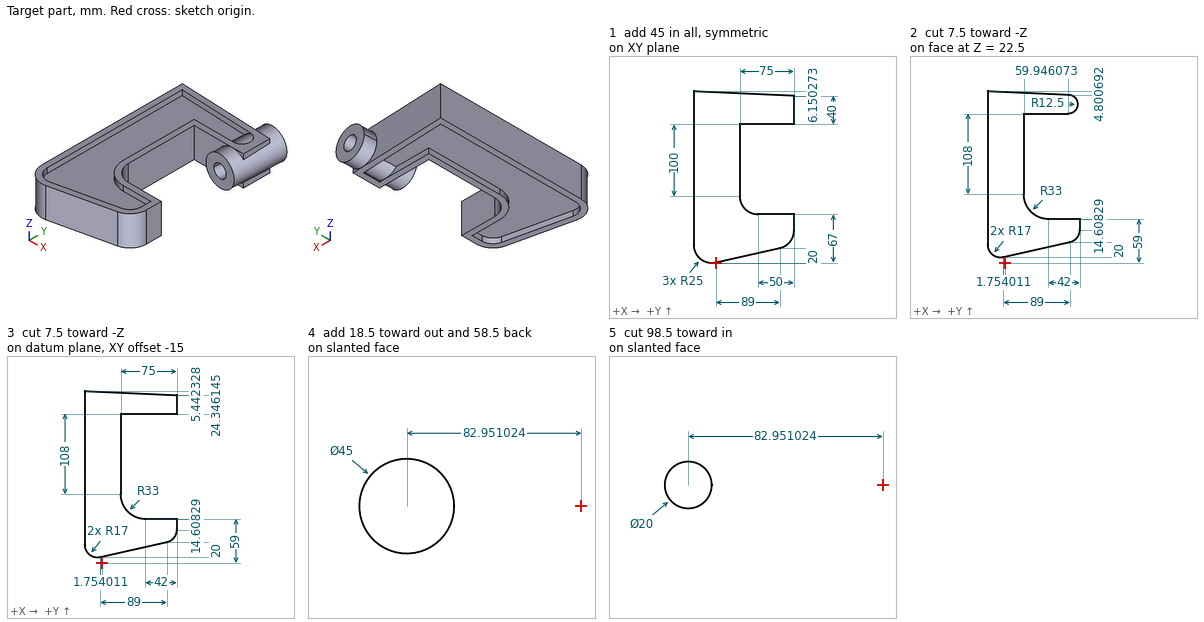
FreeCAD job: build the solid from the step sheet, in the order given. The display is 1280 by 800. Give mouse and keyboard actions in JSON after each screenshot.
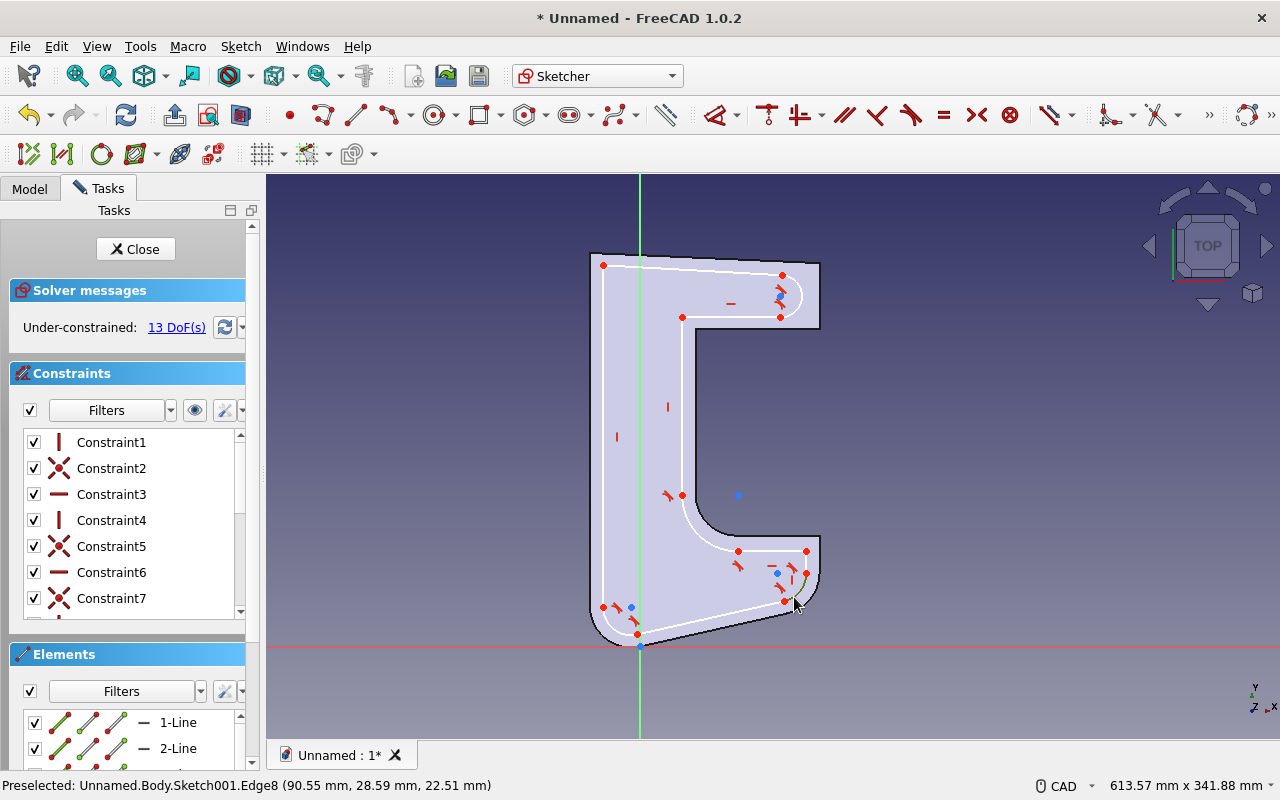
{"action": "left_click", "coordinate": [607, 622]}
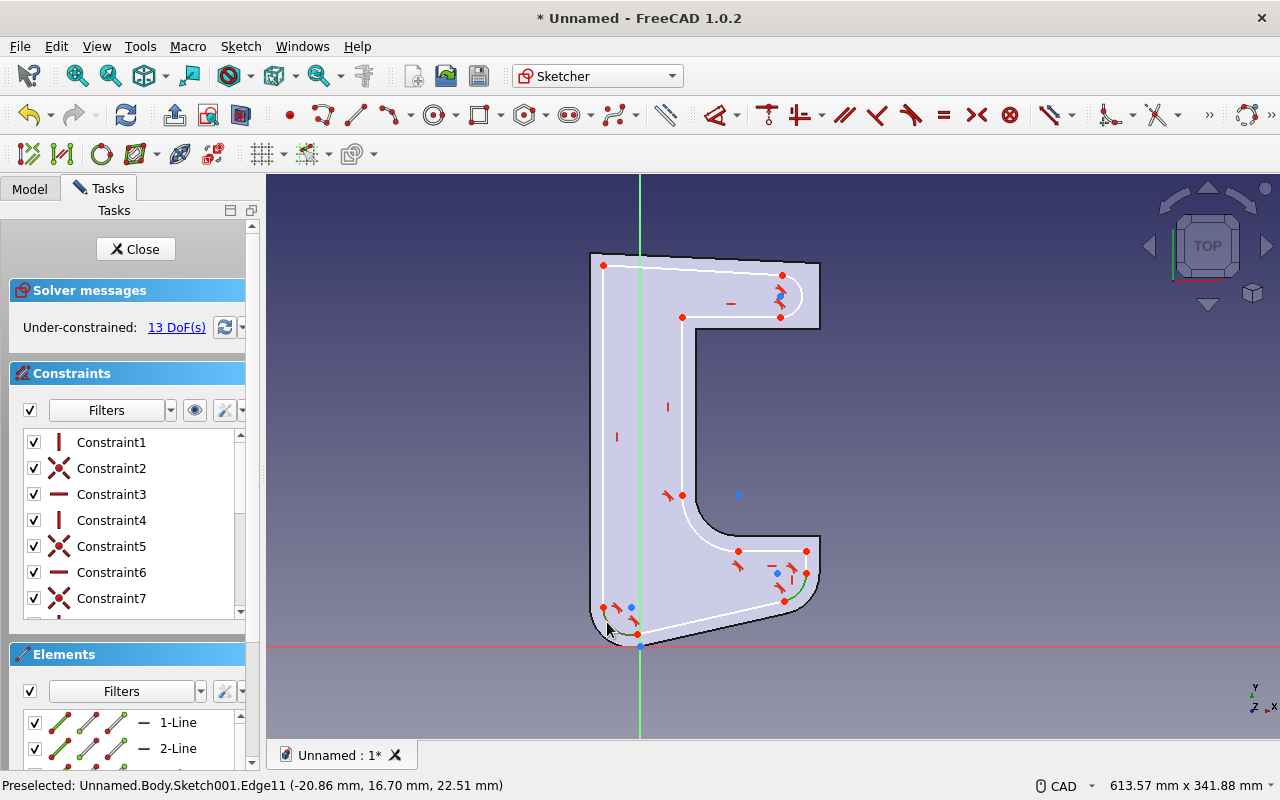
{"action": "left_click", "coordinate": [944, 116]}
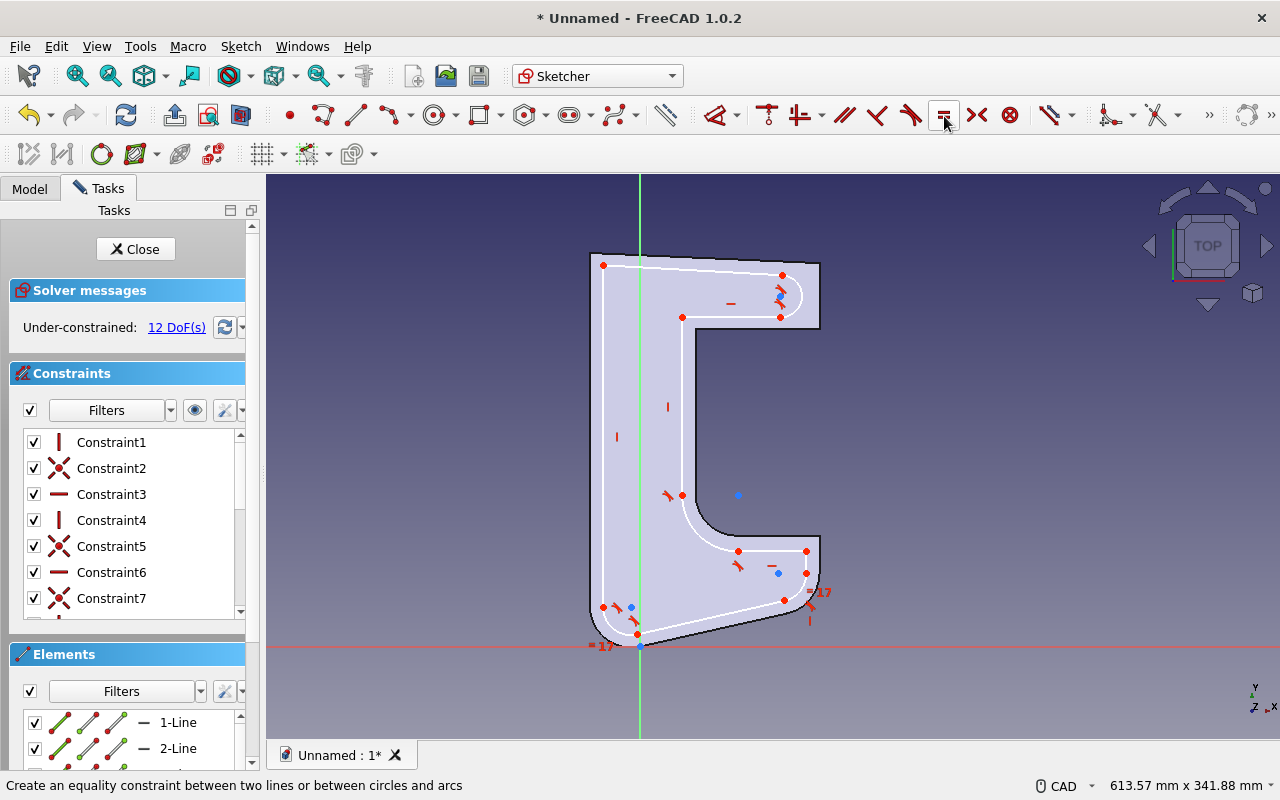
{"action": "left_click", "coordinate": [714, 116]}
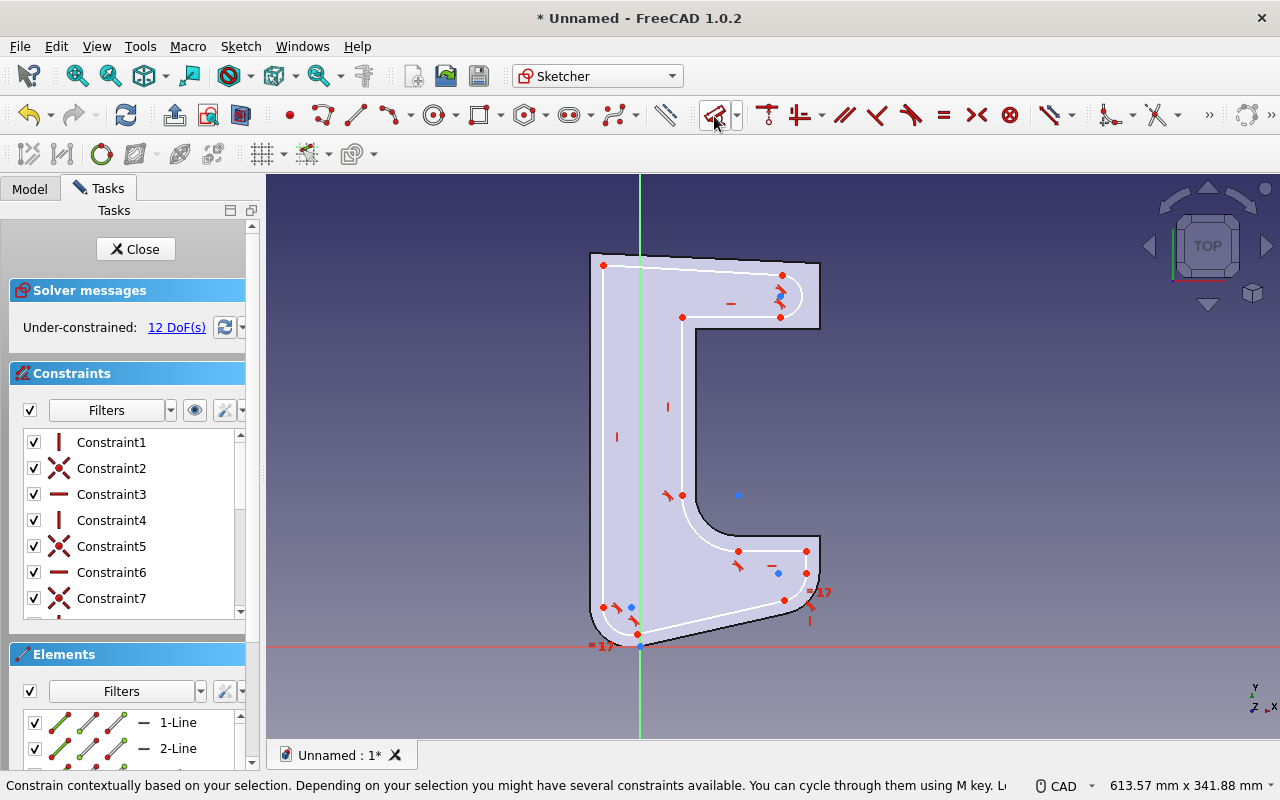
{"action": "scroll", "coordinate": [795, 596], "scroll_direction": "up", "scroll_amount": 2}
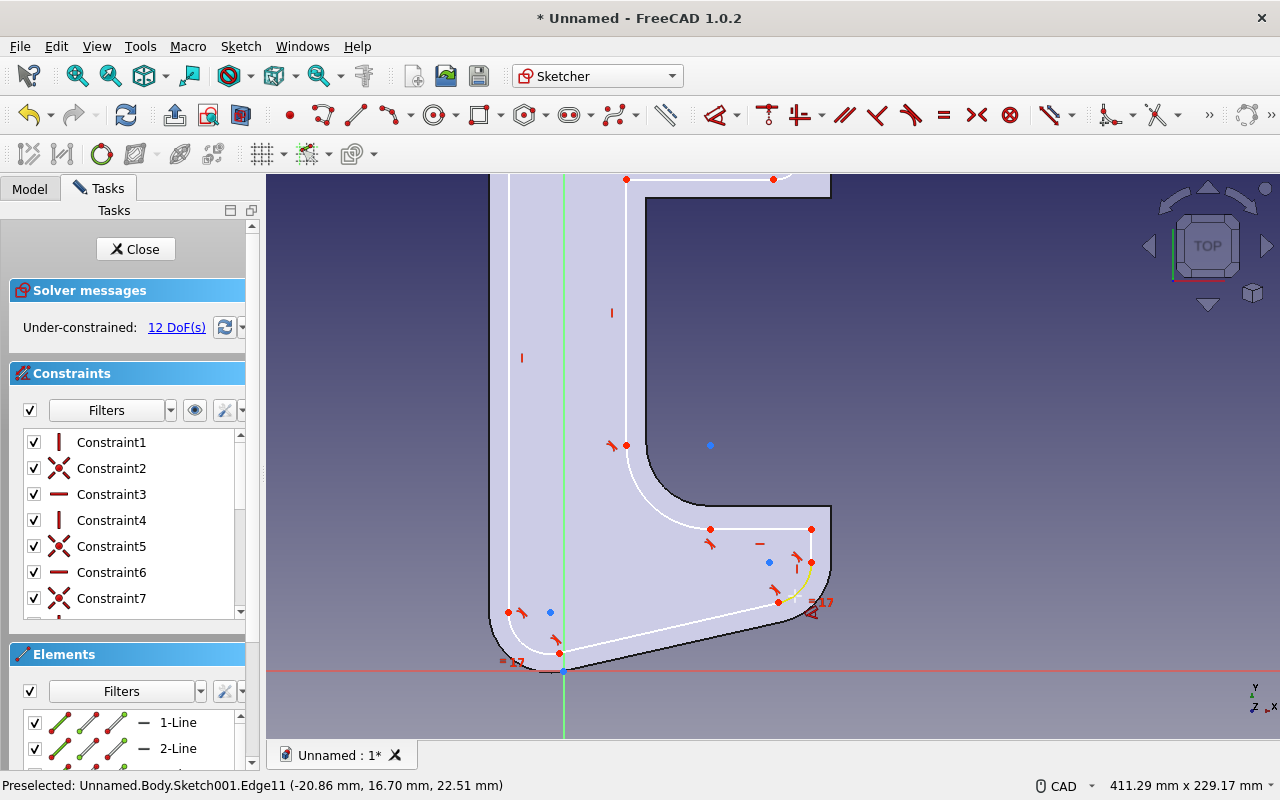
{"action": "left_click", "coordinate": [794, 596]}
{"action": "left_click", "coordinate": [813, 622]}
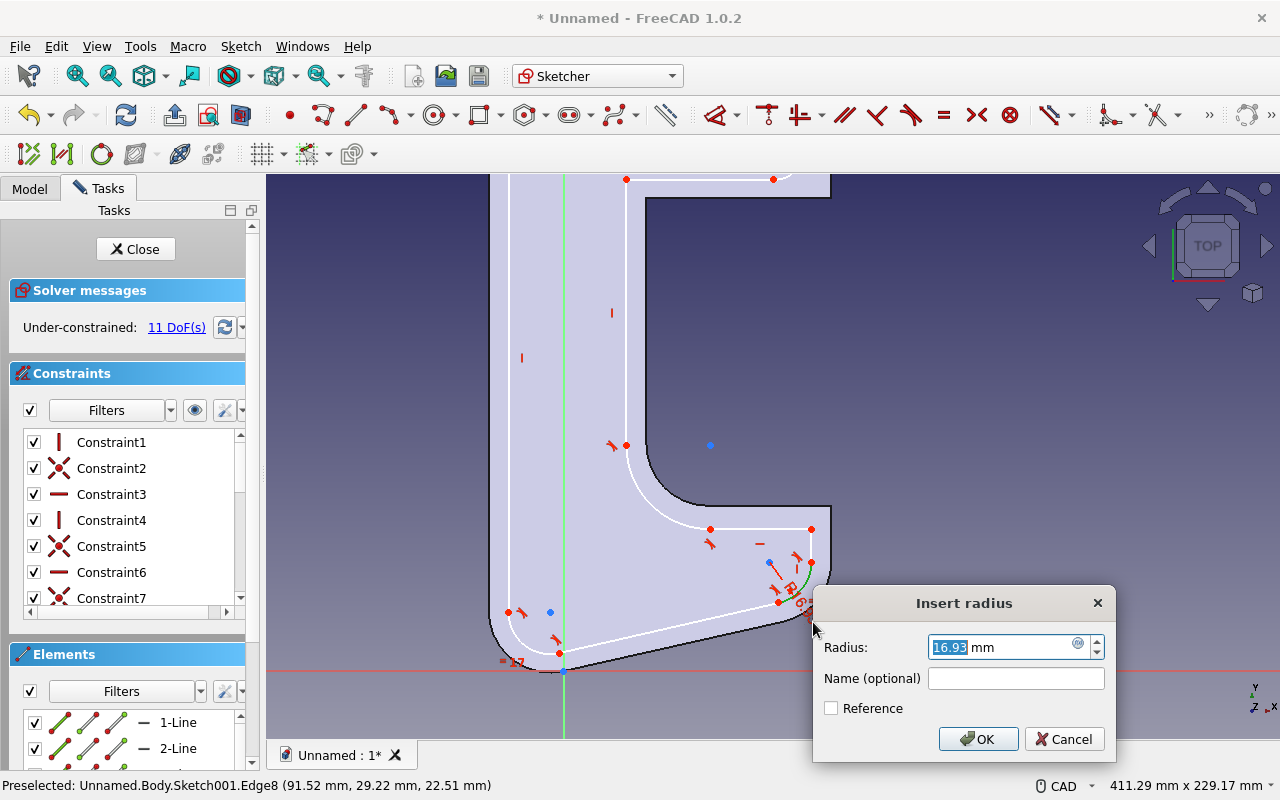
{"action": "type", "text": "17"}
{"action": "key", "text": "Return"}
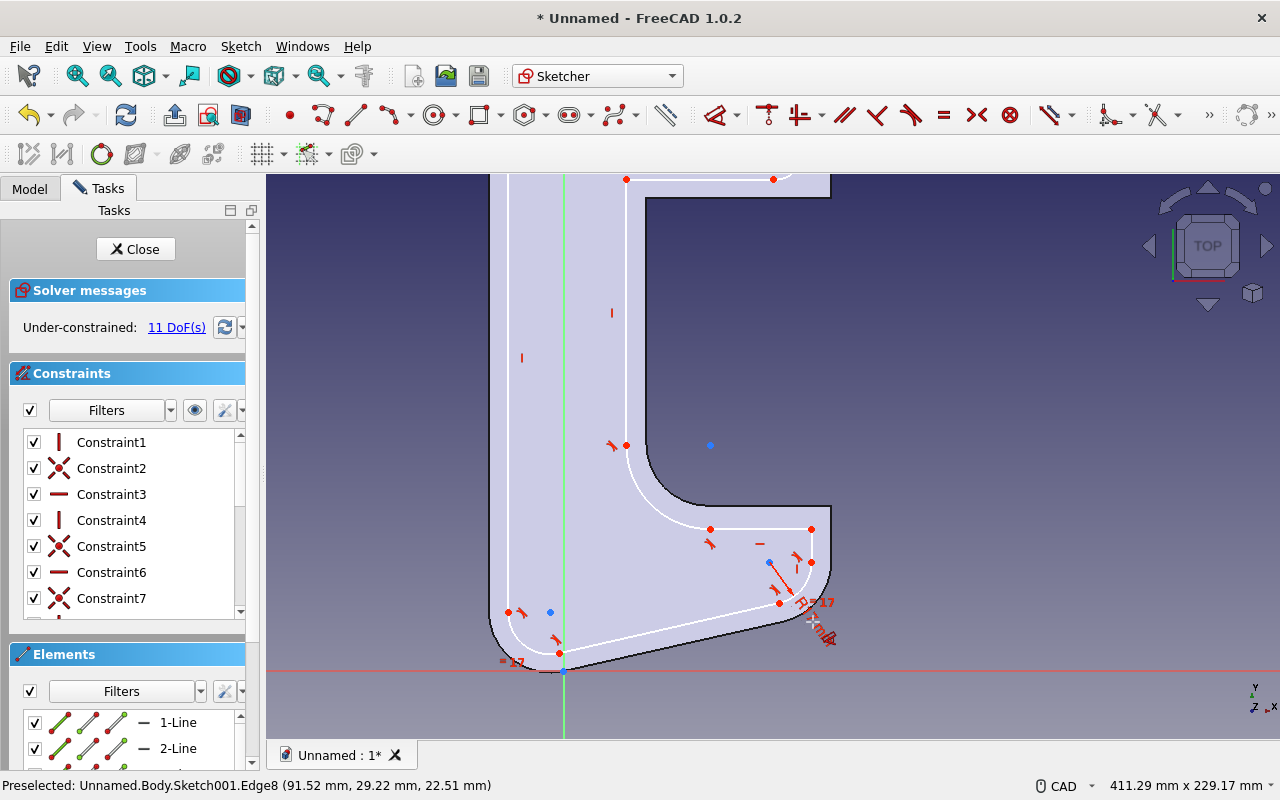
{"action": "left_click", "coordinate": [636, 483]}
{"action": "left_click", "coordinate": [607, 497]}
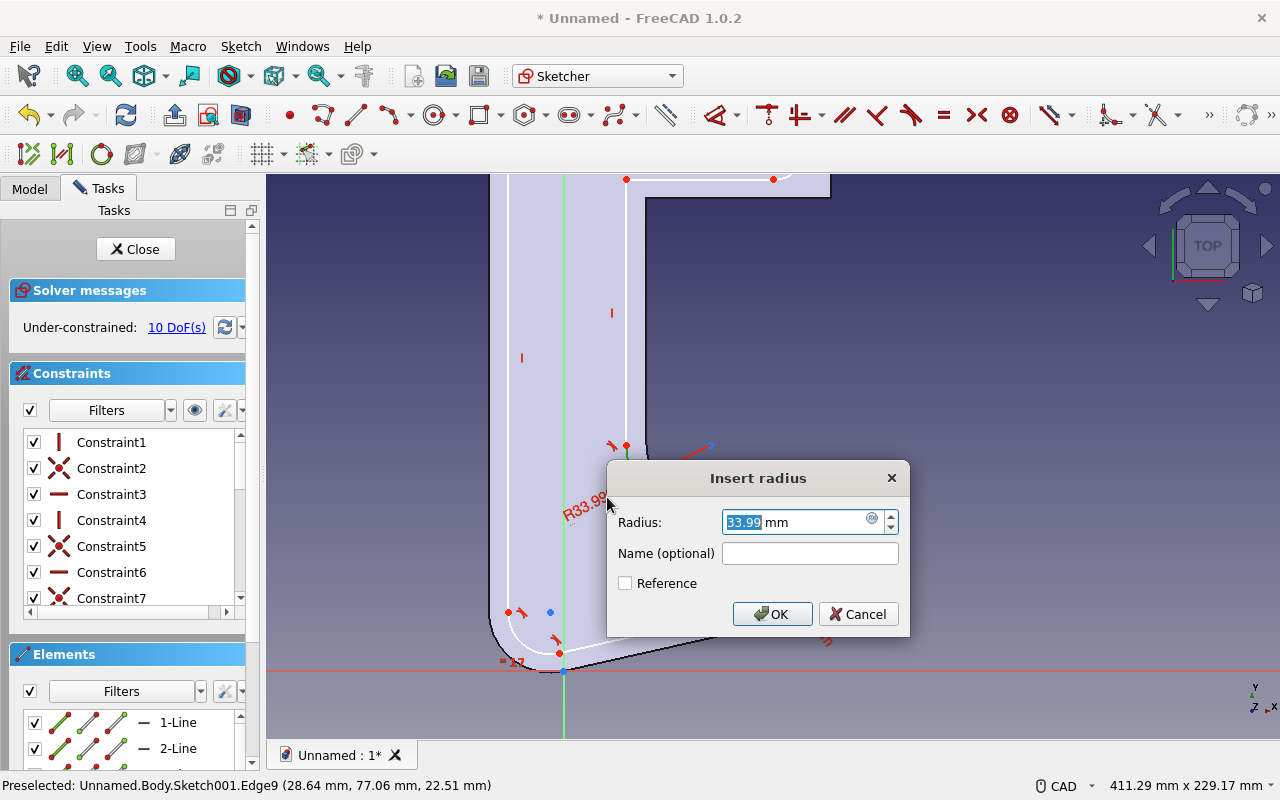
{"action": "type", "text": "33"}
{"action": "key", "text": "Return"}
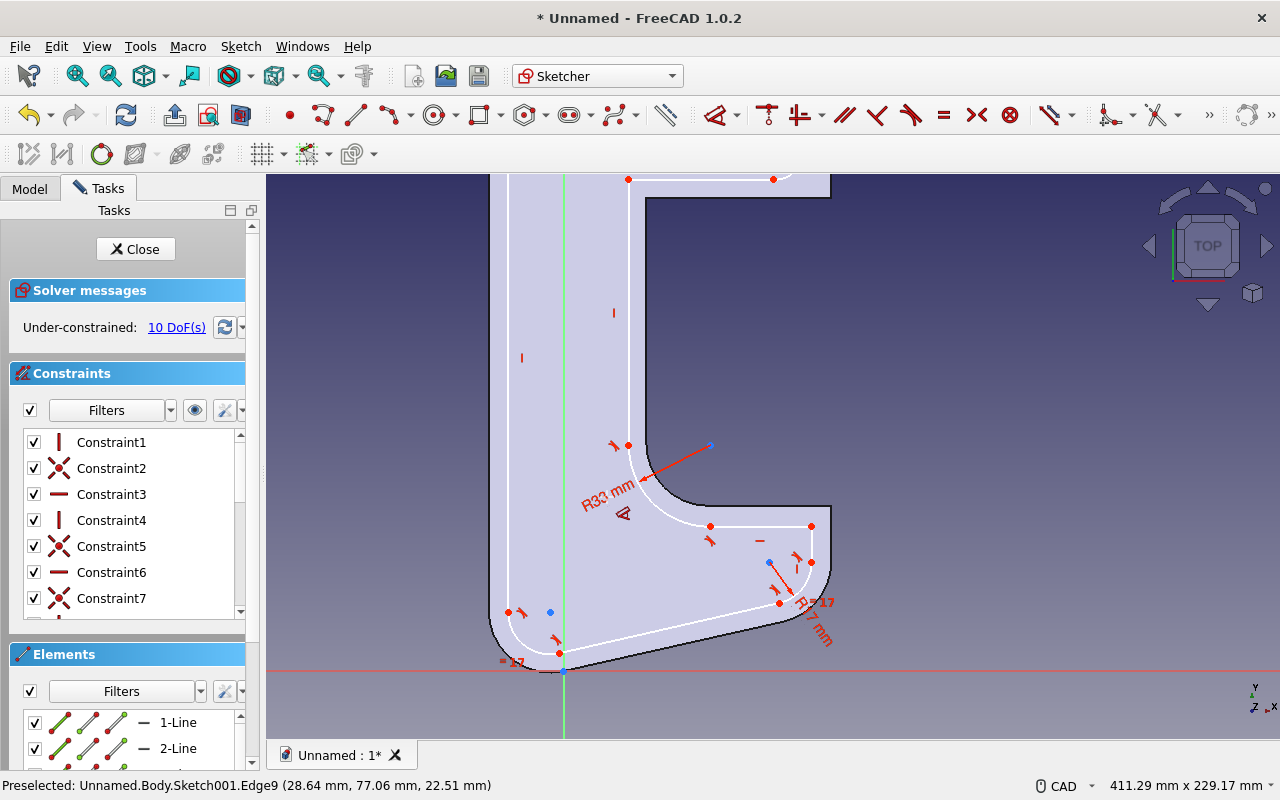
{"action": "scroll", "coordinate": [795, 596], "scroll_direction": "down", "scroll_amount": 2}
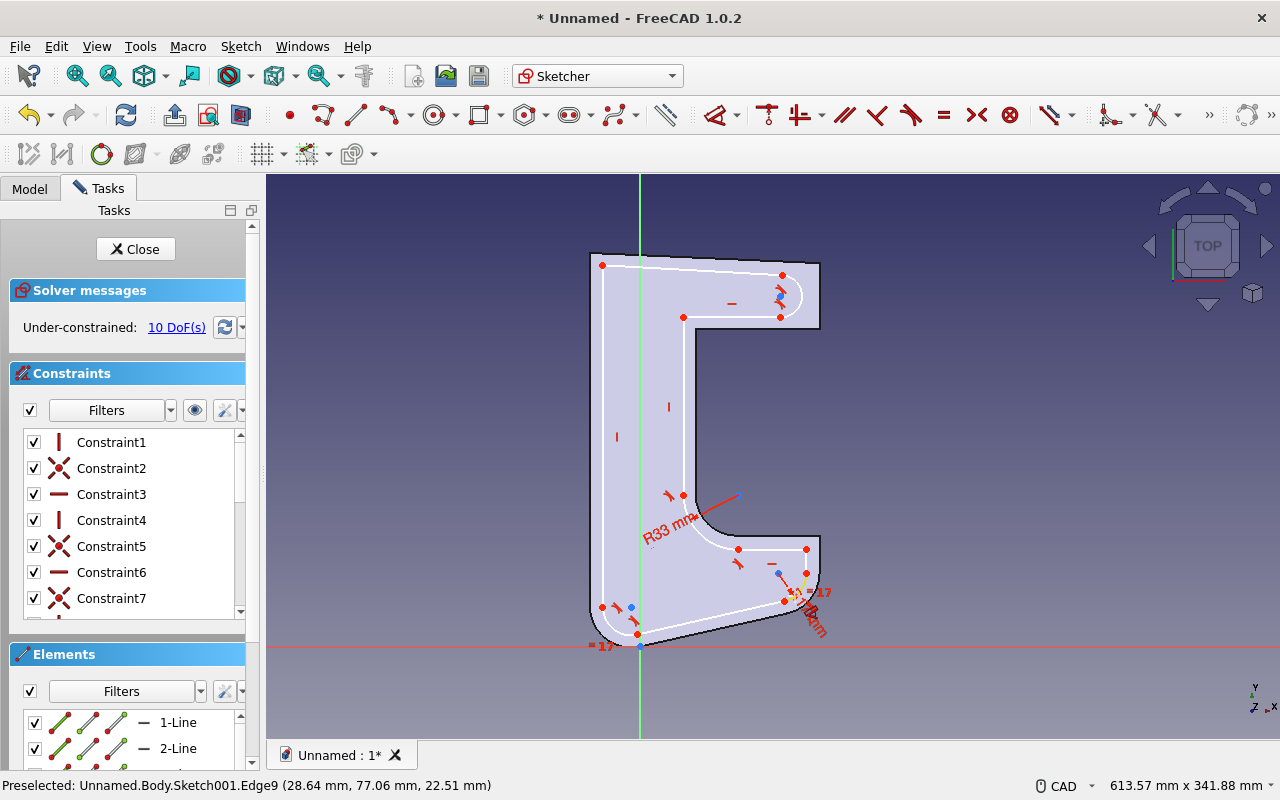
{"action": "scroll", "coordinate": [798, 309], "scroll_direction": "up", "scroll_amount": 4}